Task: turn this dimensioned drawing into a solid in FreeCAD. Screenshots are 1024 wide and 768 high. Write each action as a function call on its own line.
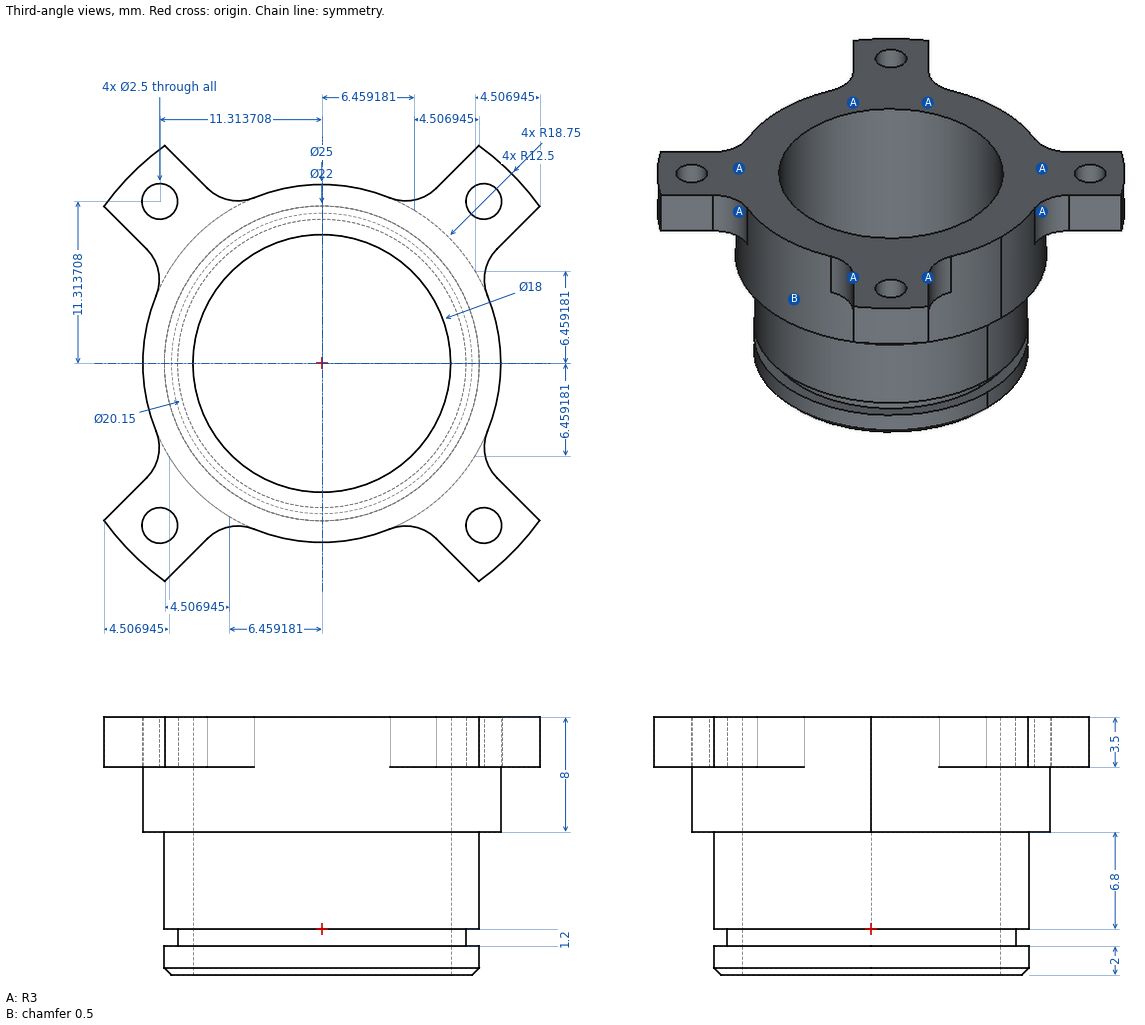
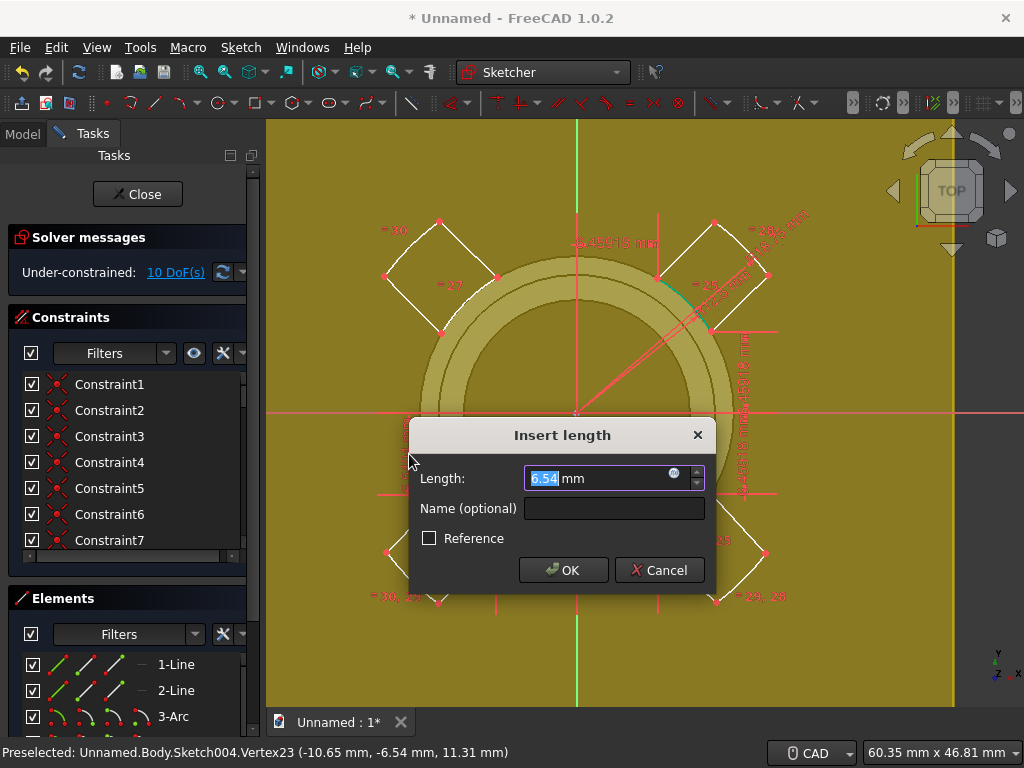
text(6.459181)
key(Return)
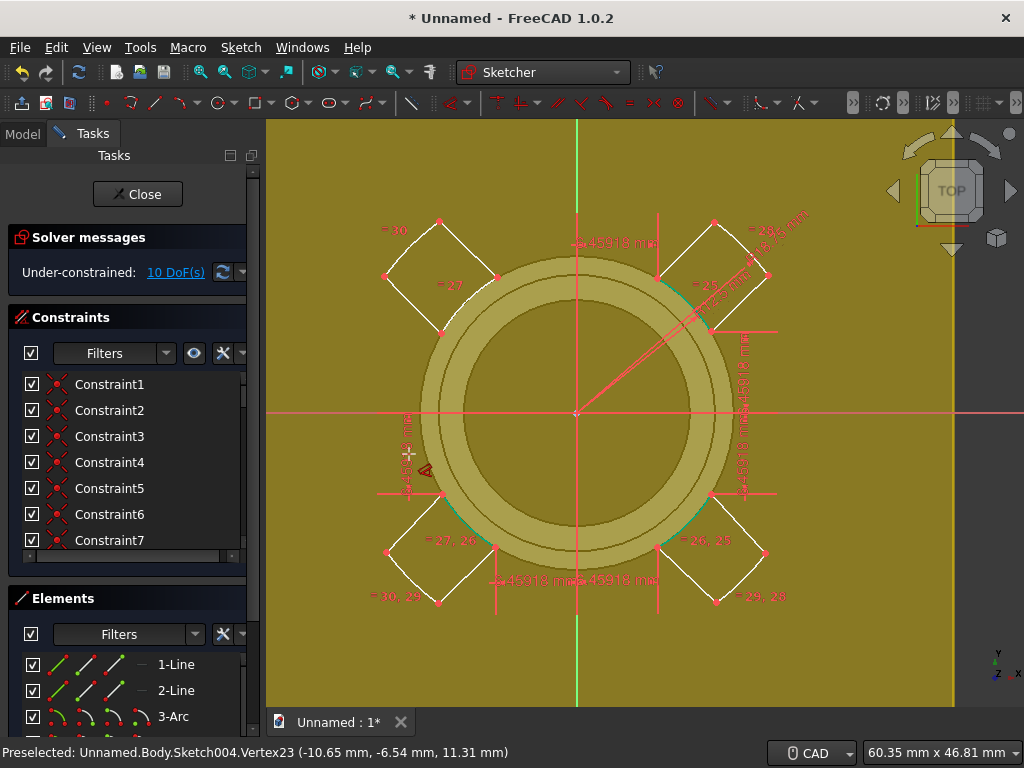
click(441, 334)
click(407, 373)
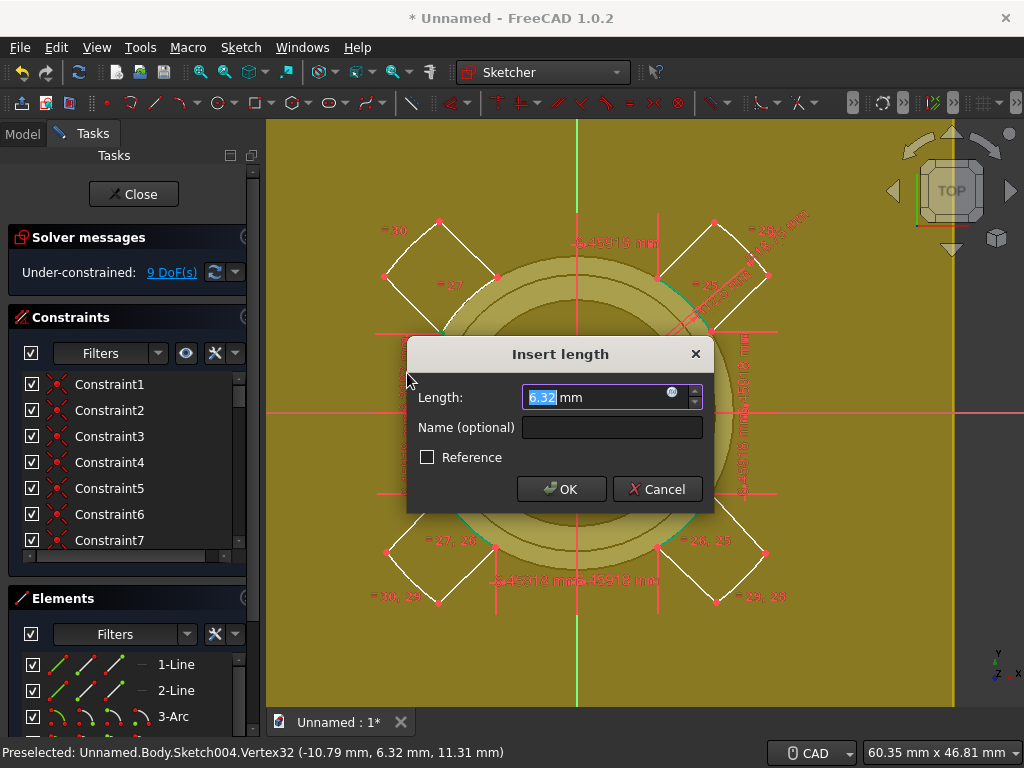
text(6.459181)
key(Return)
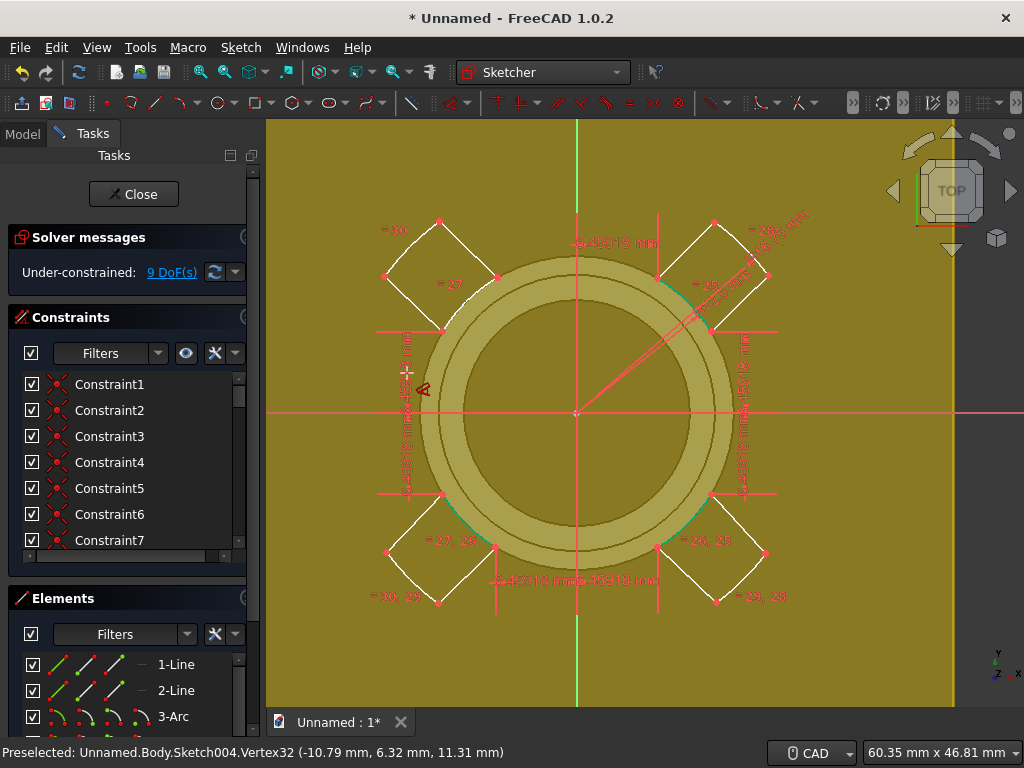
click(497, 278)
click(537, 244)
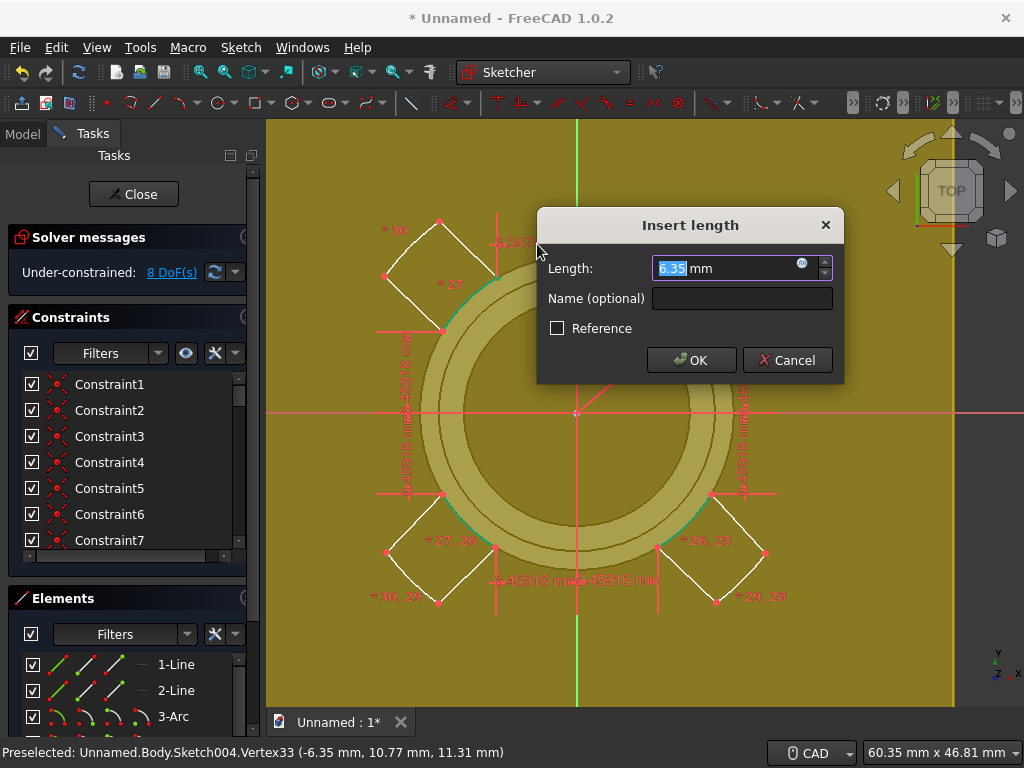
text(6.459181)
key(Return)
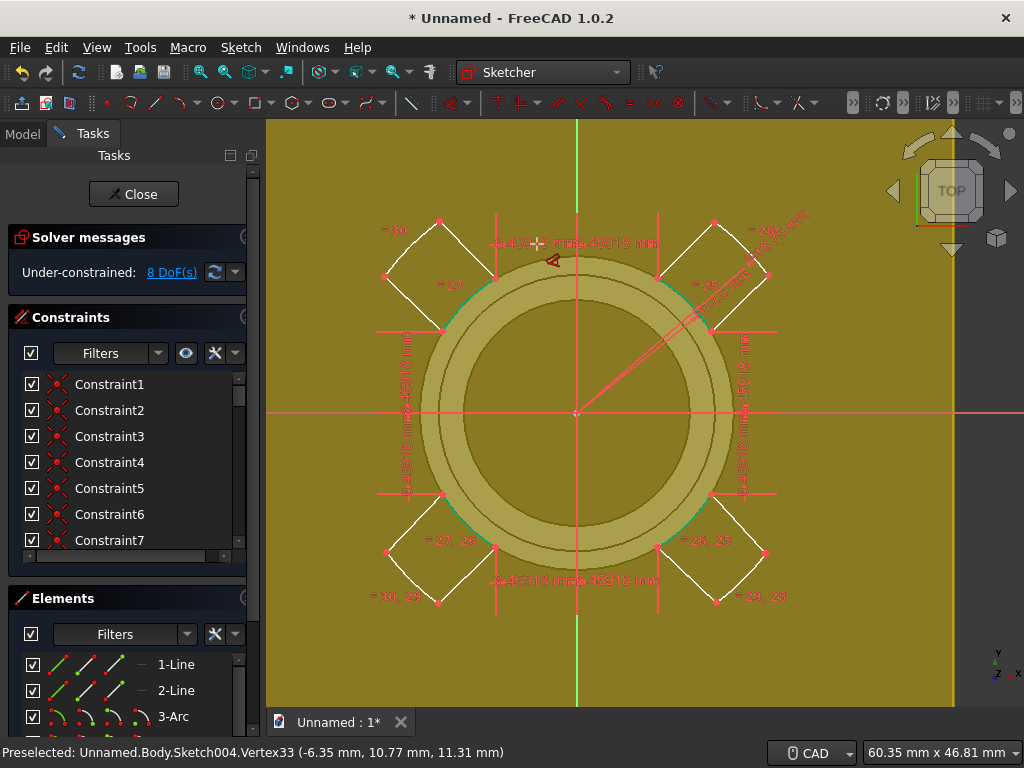
click(698, 239)
click(686, 188)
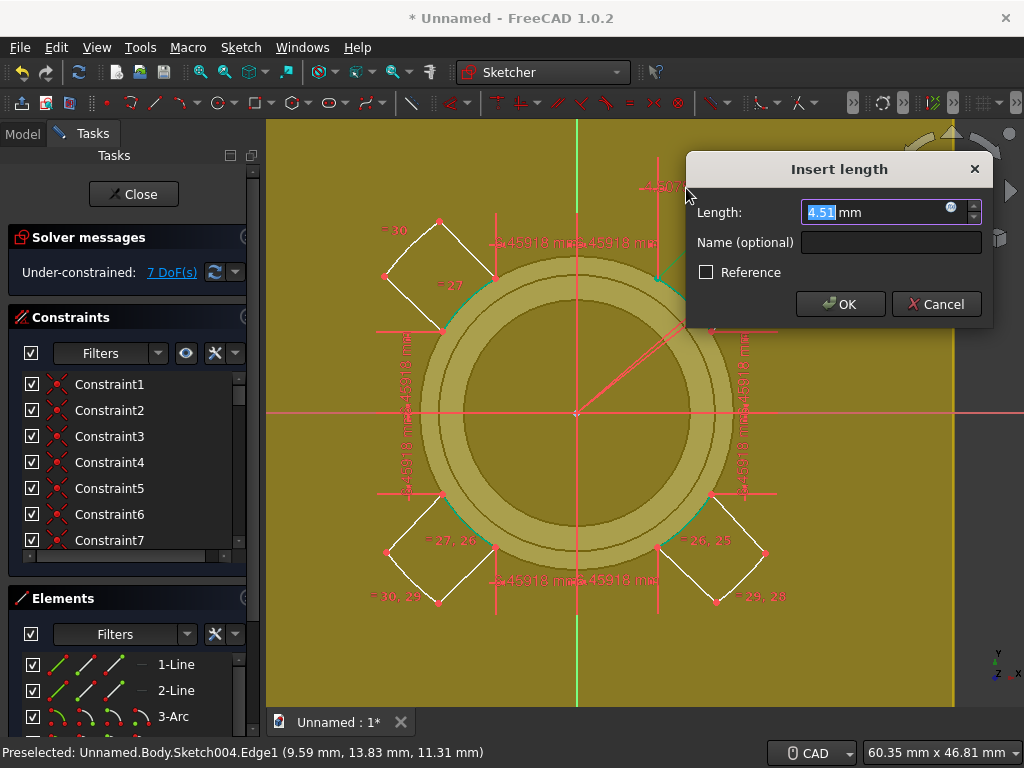
text(4.506945)
key(Return)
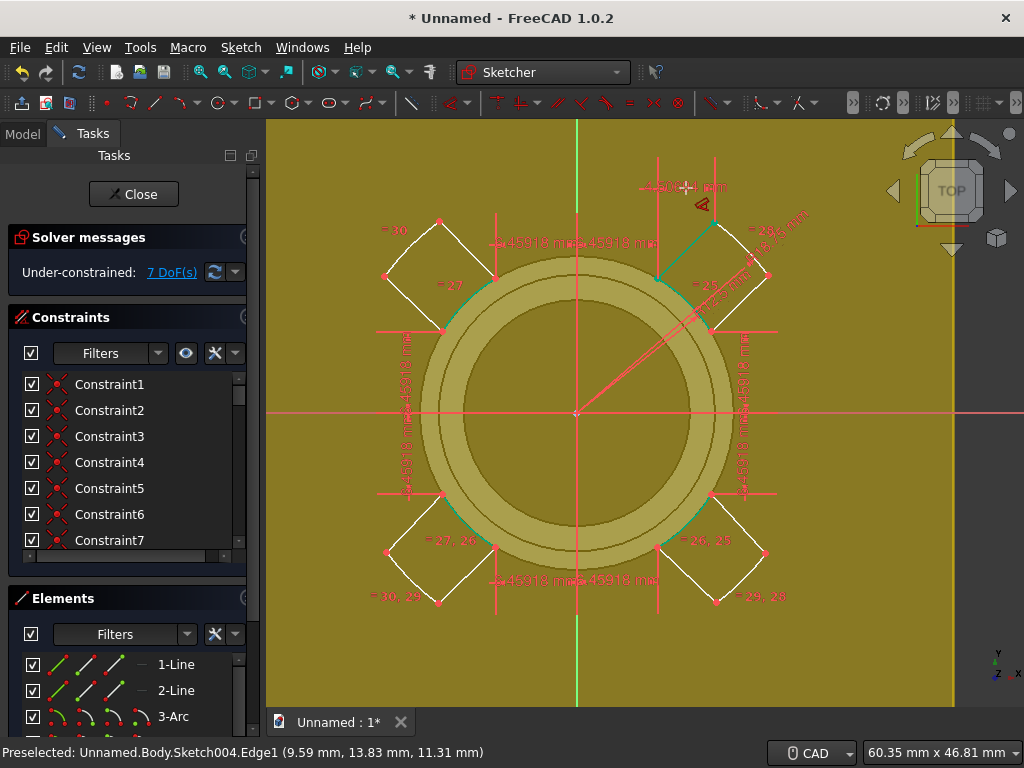
click(728, 315)
click(760, 194)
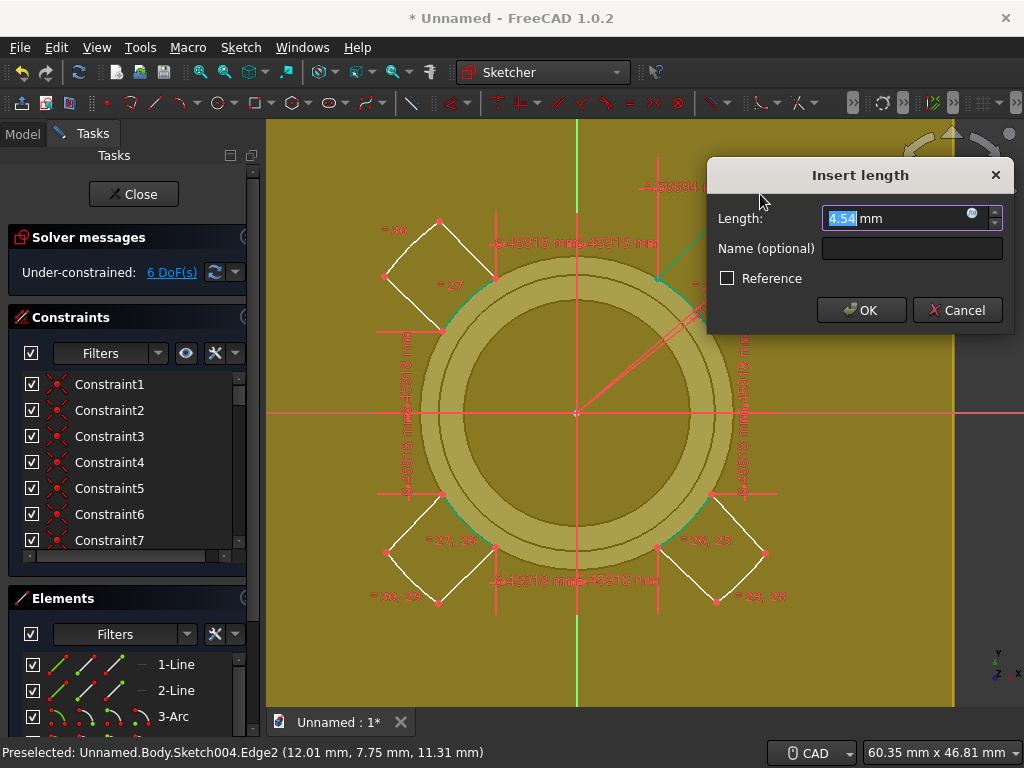
text(4.506945)
key(Return)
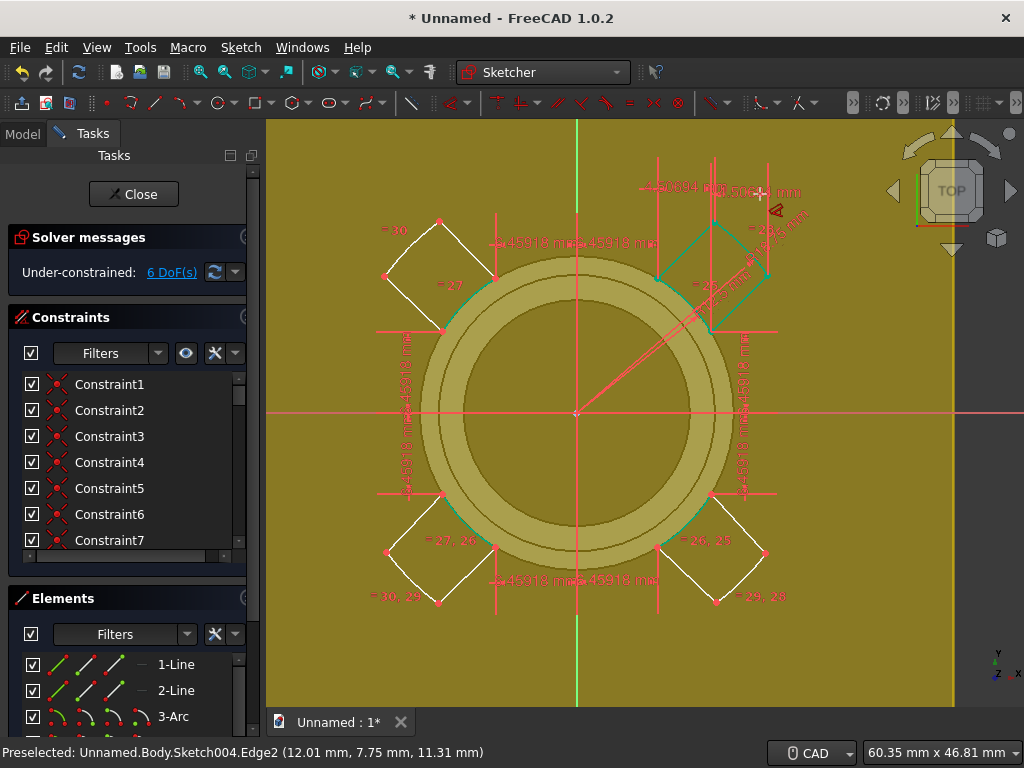
click(749, 536)
click(758, 588)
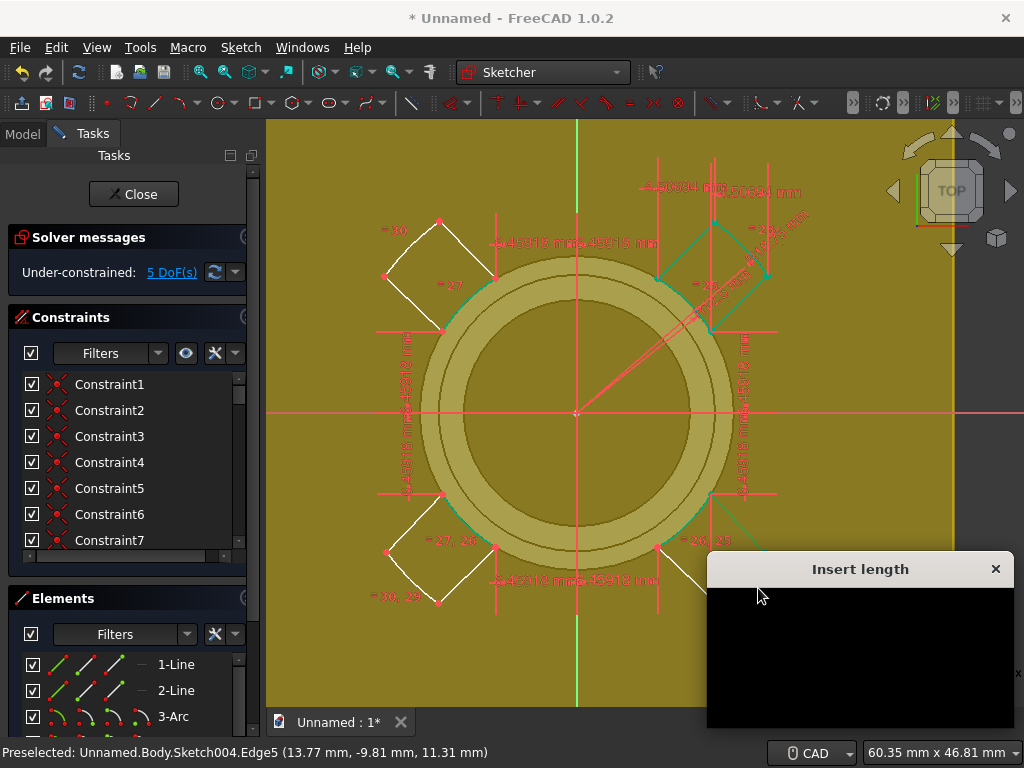
text(4.506945)
key(Return)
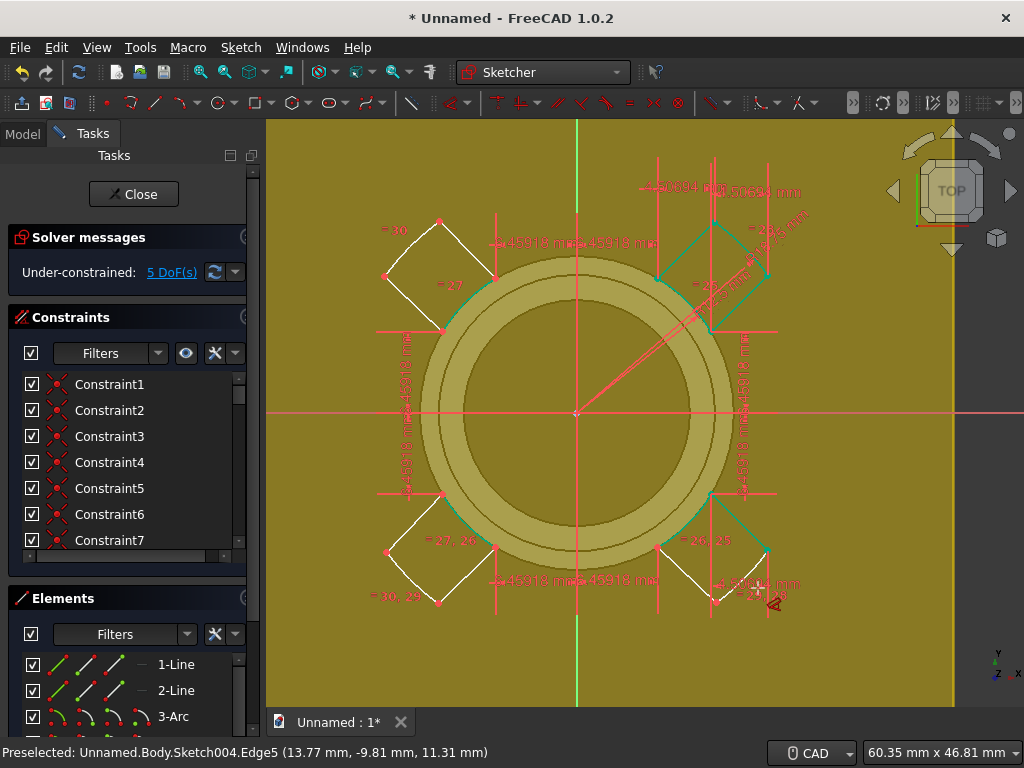
click(675, 564)
click(687, 637)